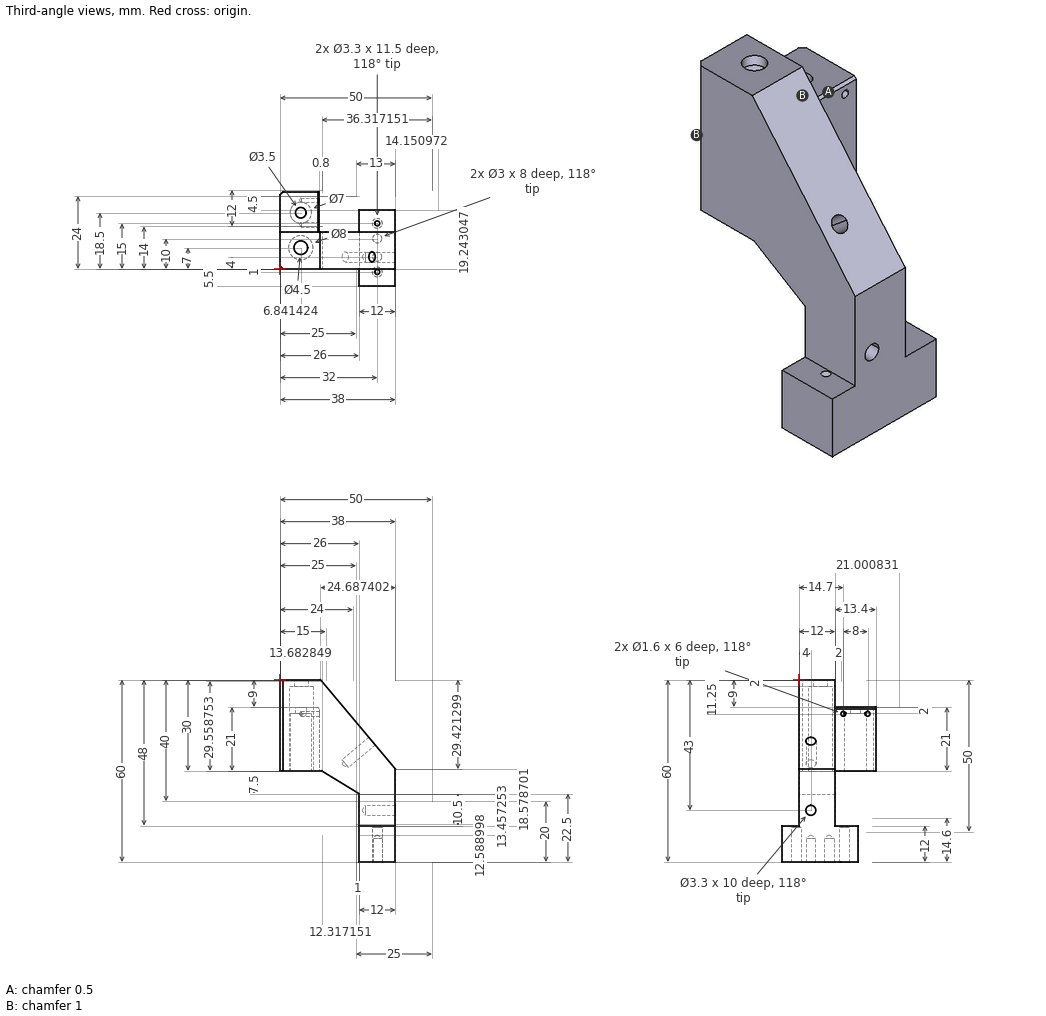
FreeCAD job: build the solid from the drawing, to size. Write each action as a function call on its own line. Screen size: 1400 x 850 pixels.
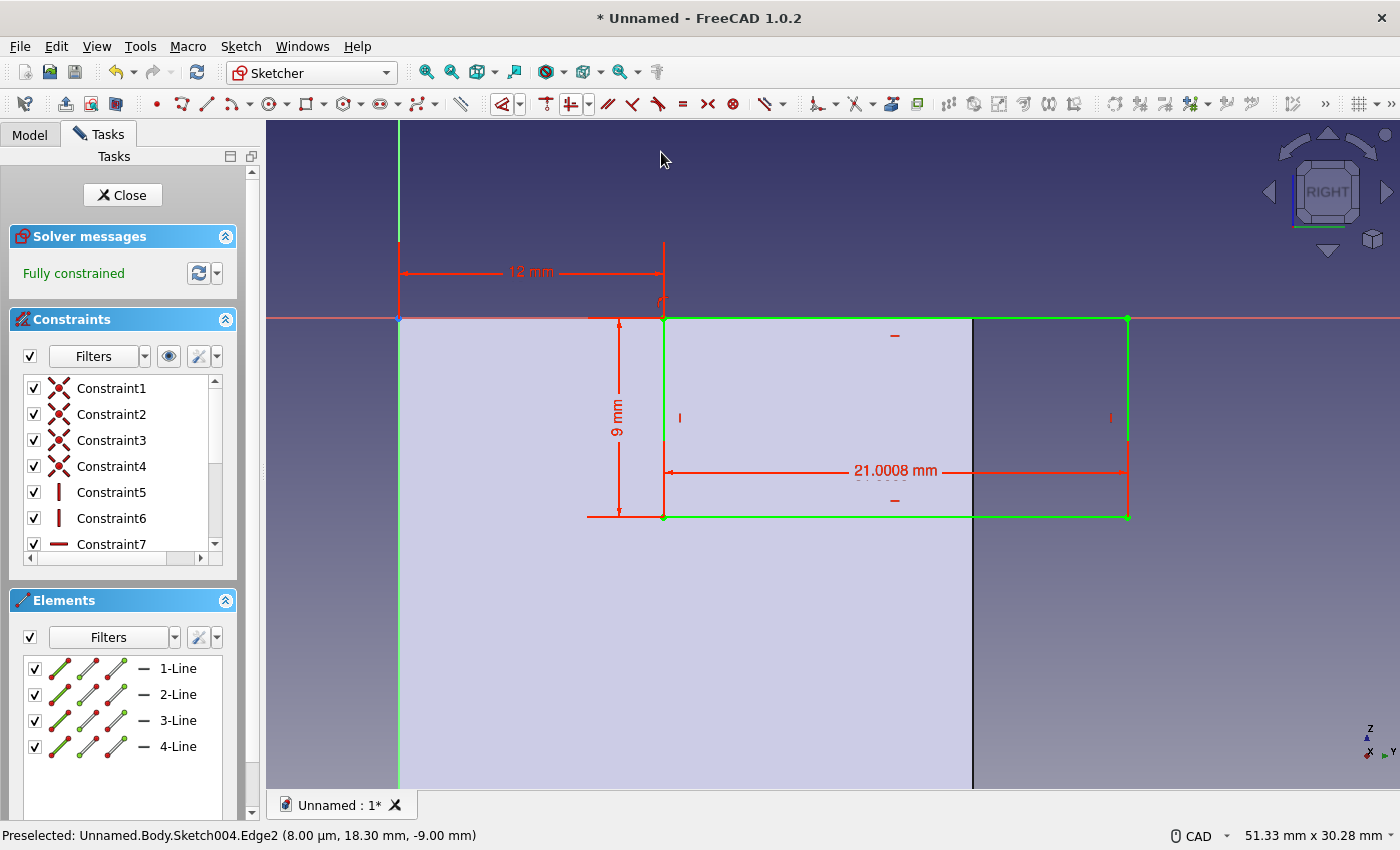
click(123, 195)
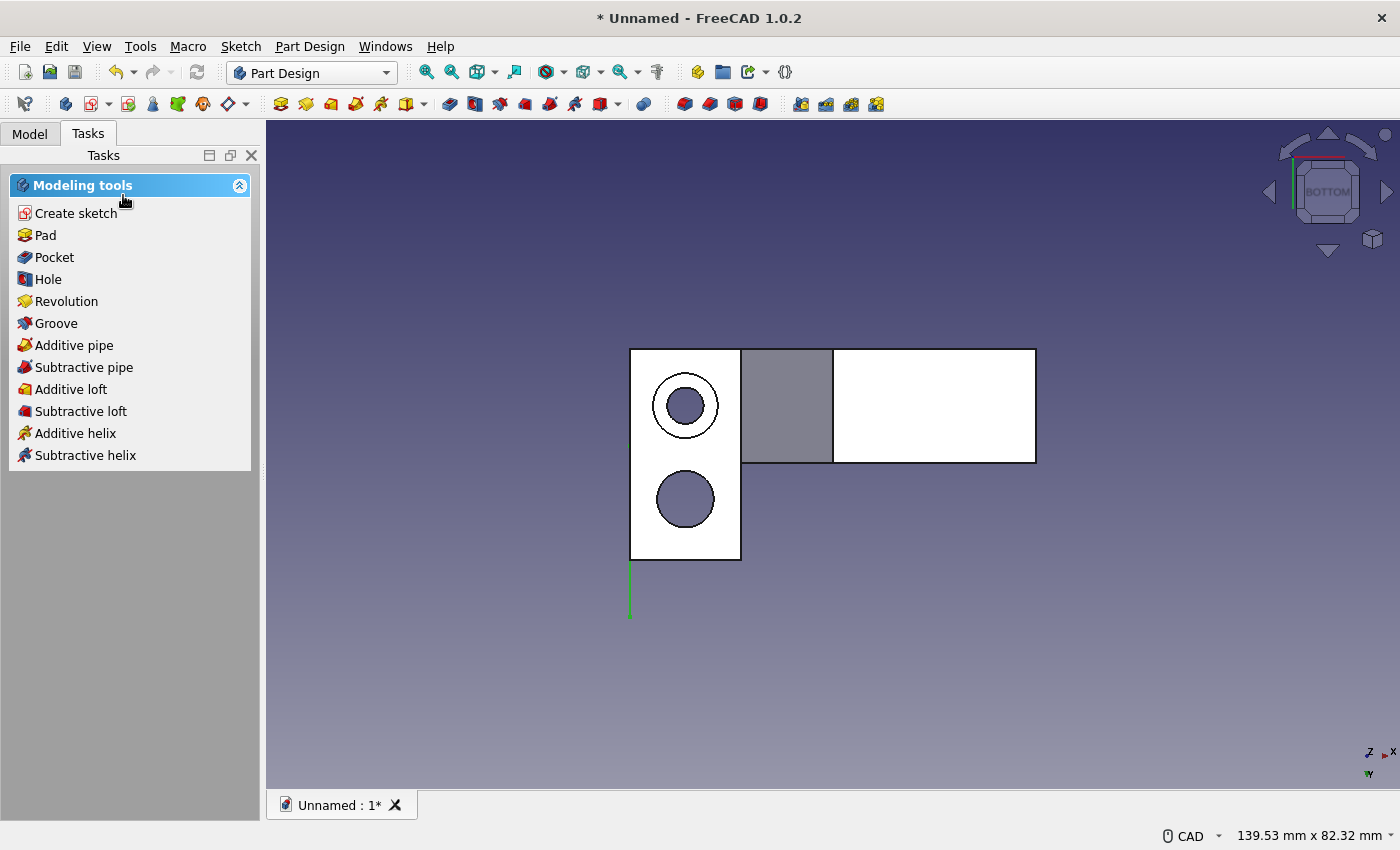
click(450, 104)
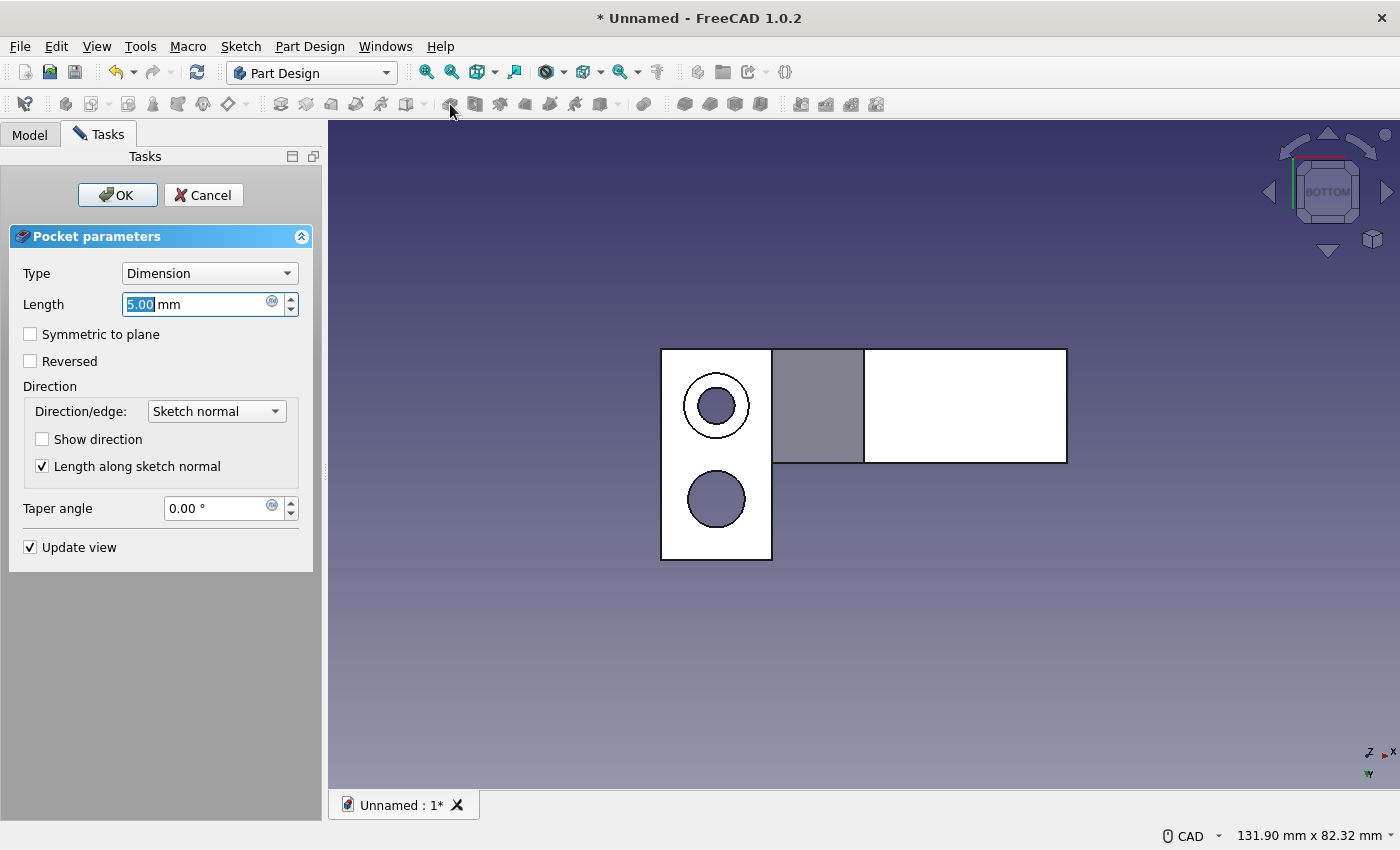
text(15)
key(Tab)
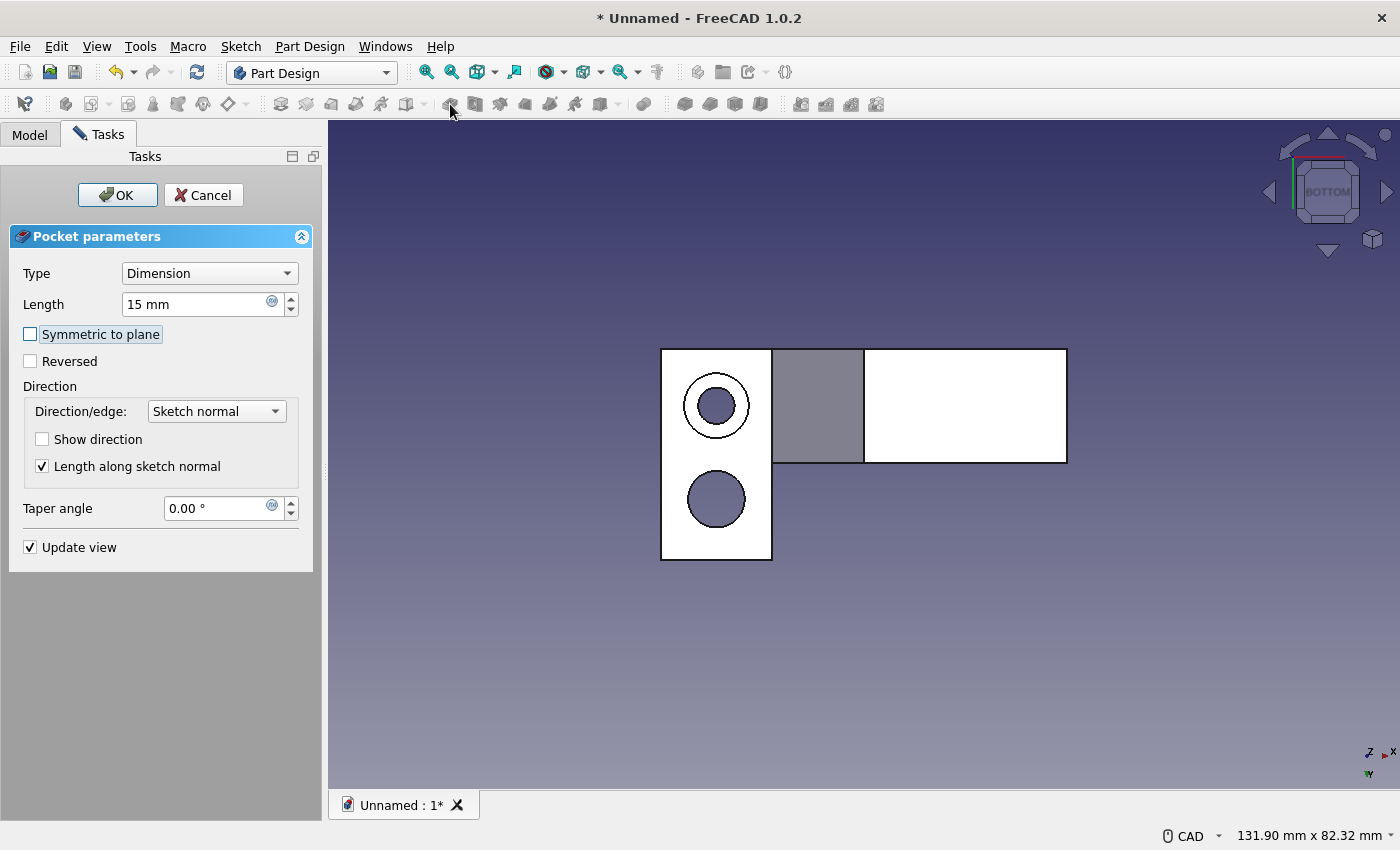
click(31, 361)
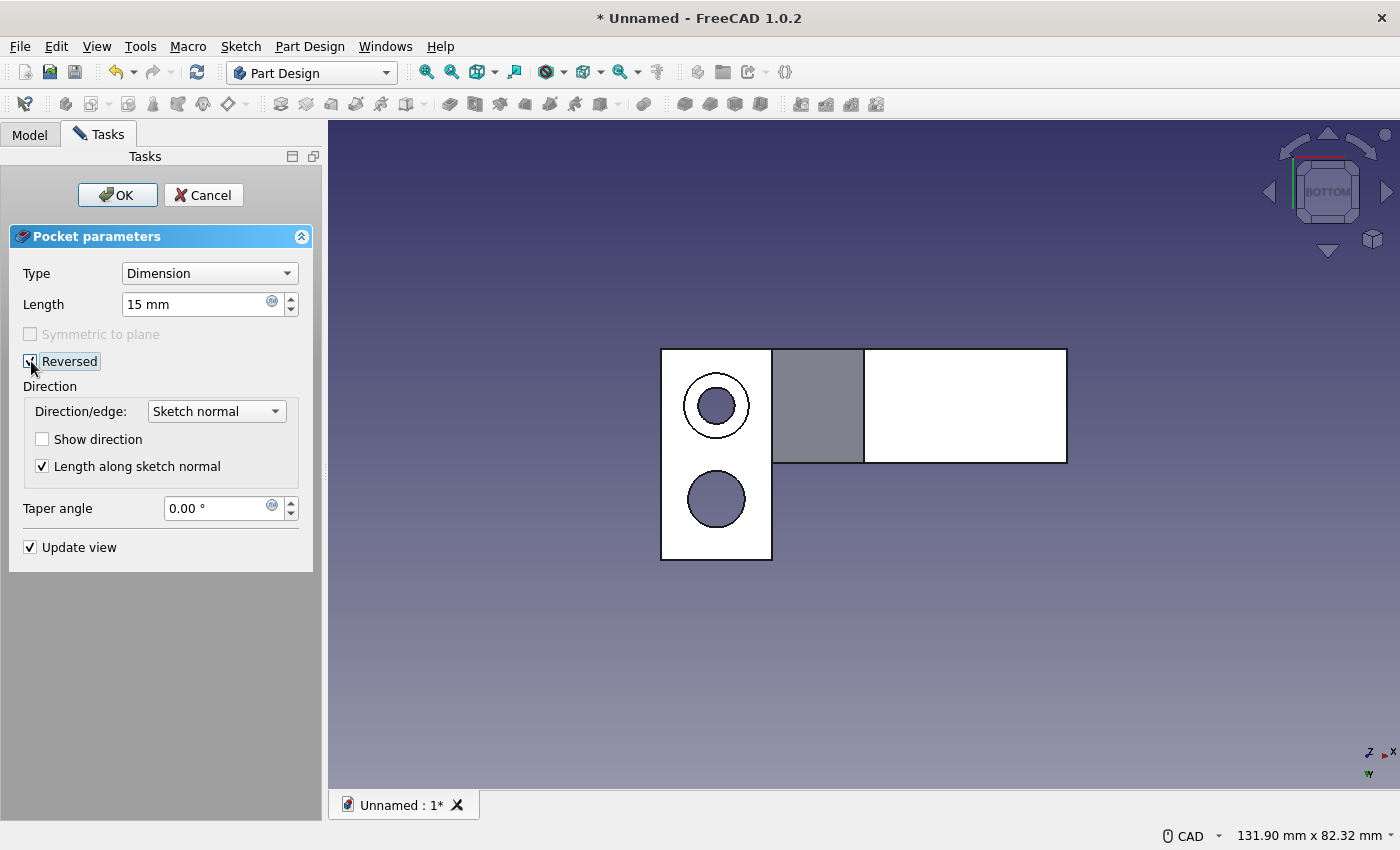
click(118, 195)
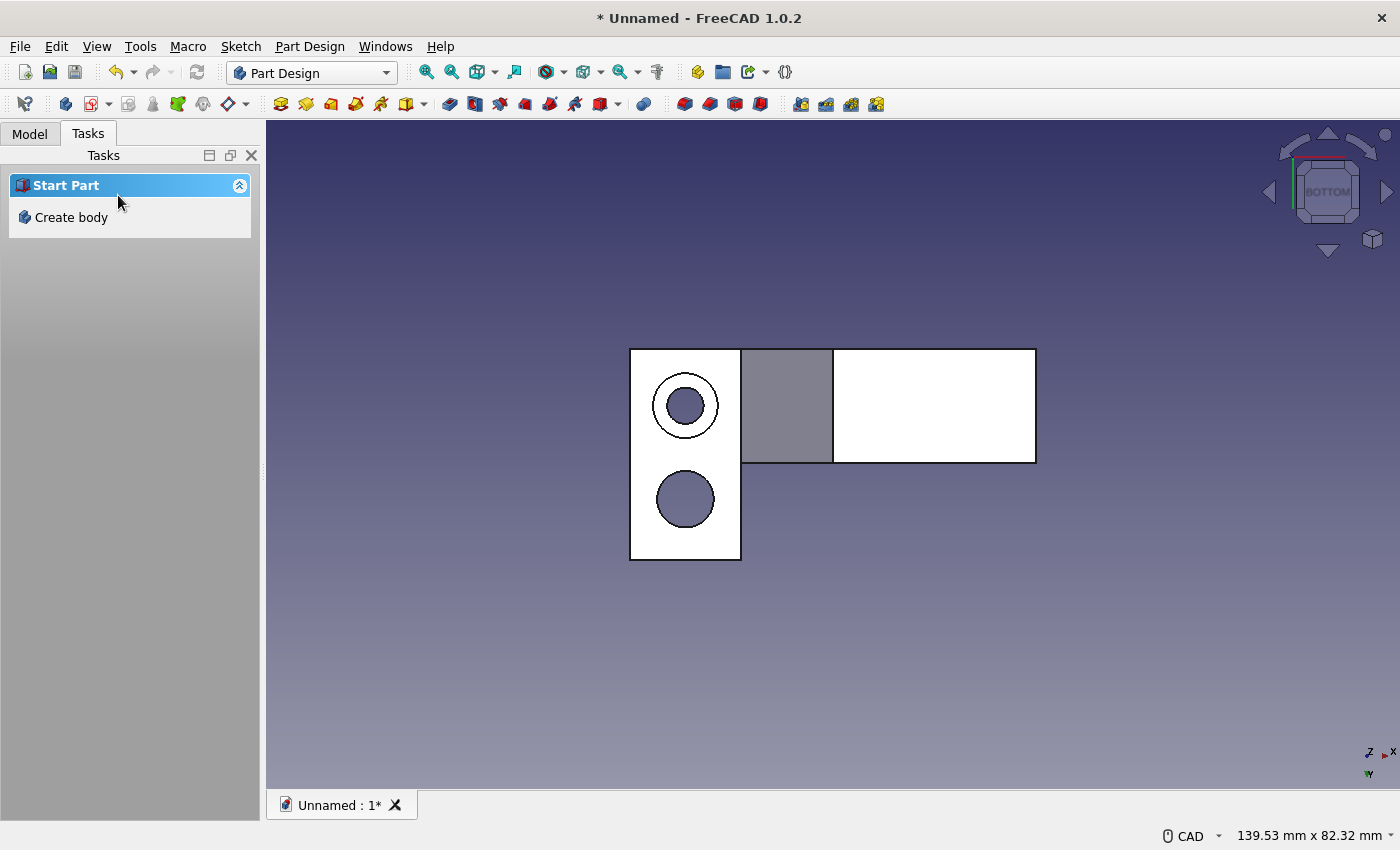
click(427, 72)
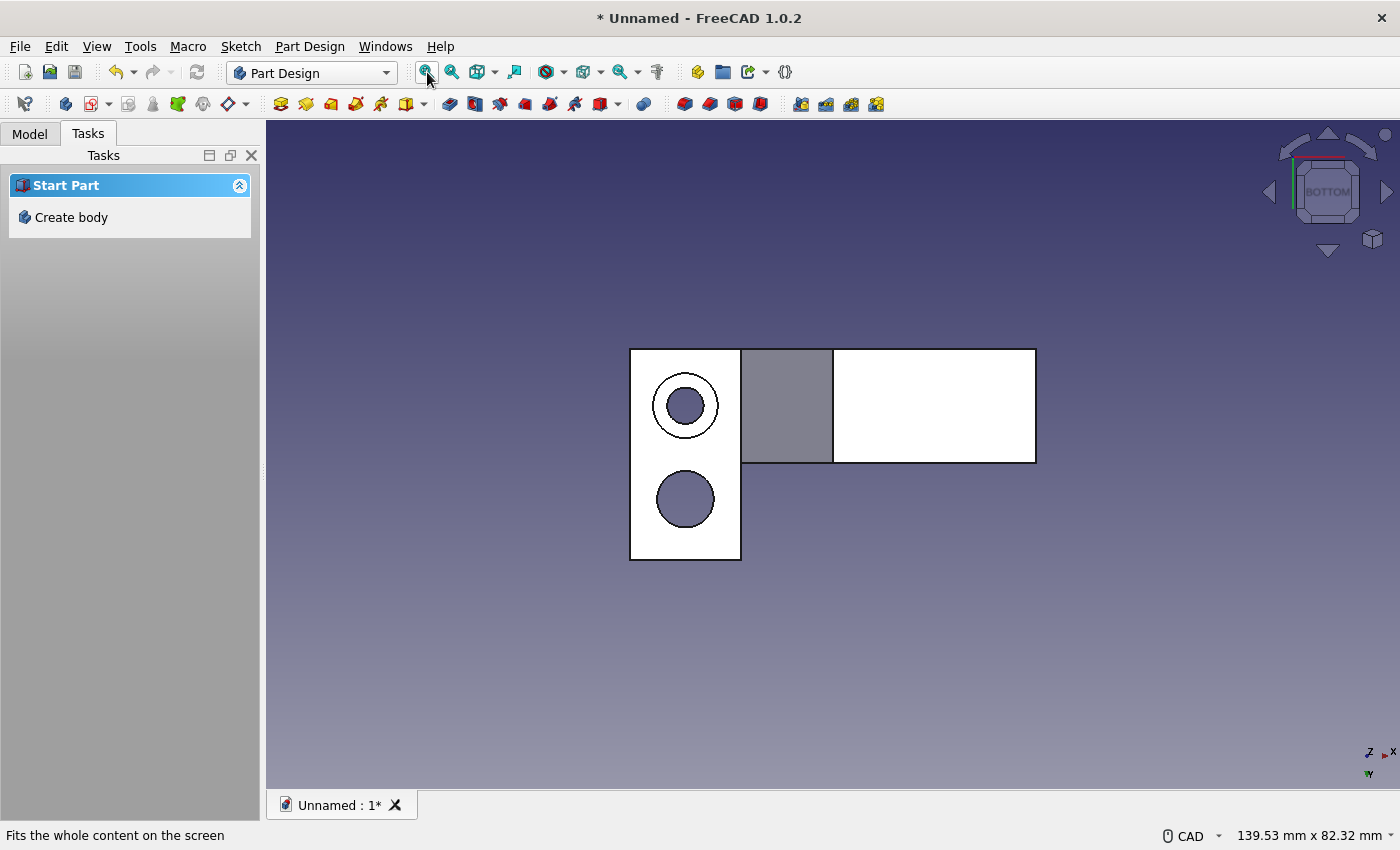
key(0)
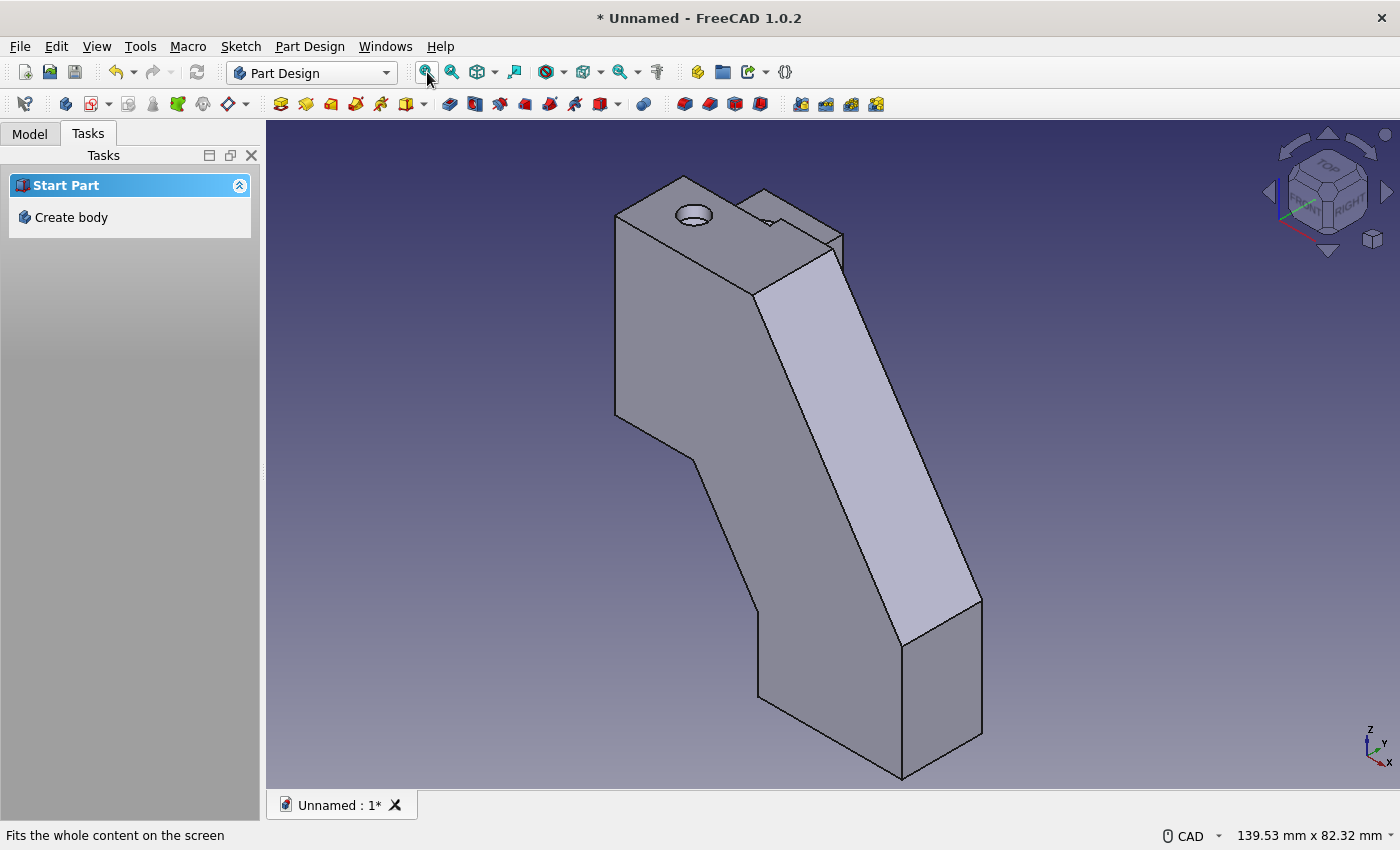
click(765, 209)